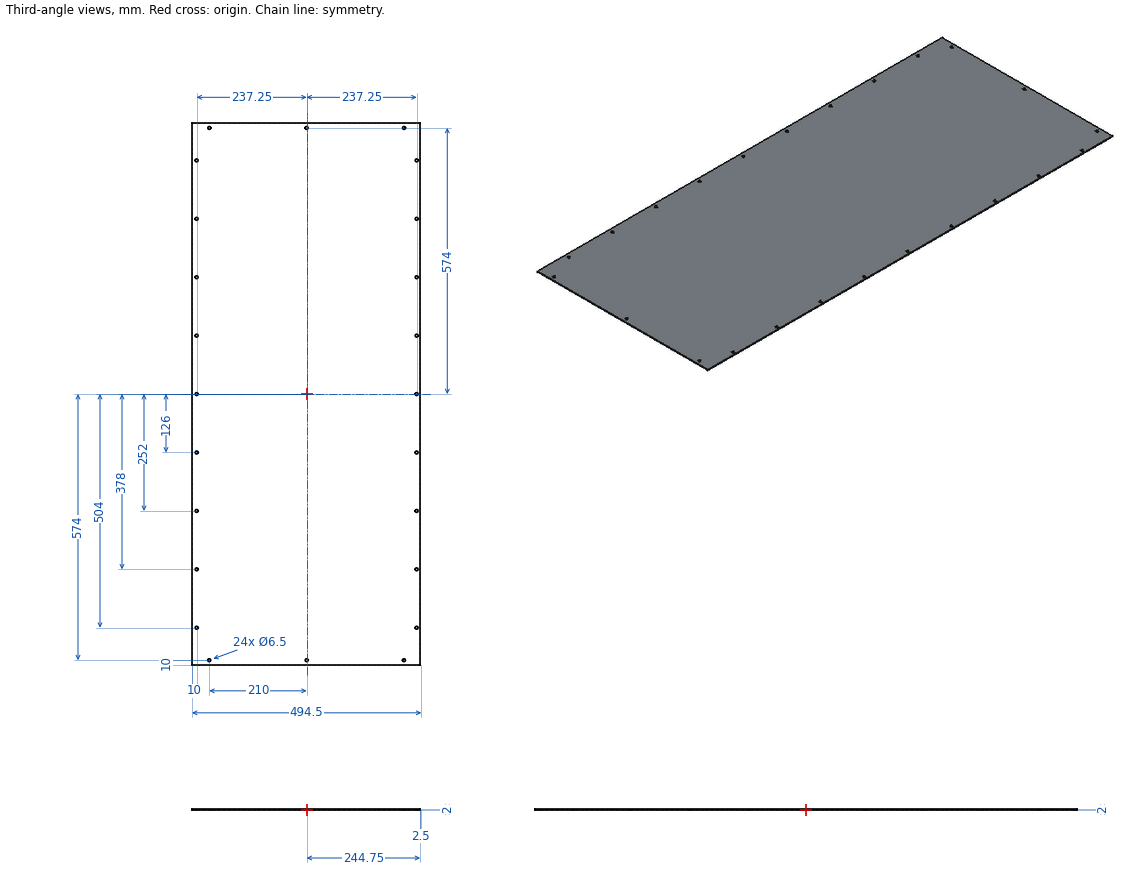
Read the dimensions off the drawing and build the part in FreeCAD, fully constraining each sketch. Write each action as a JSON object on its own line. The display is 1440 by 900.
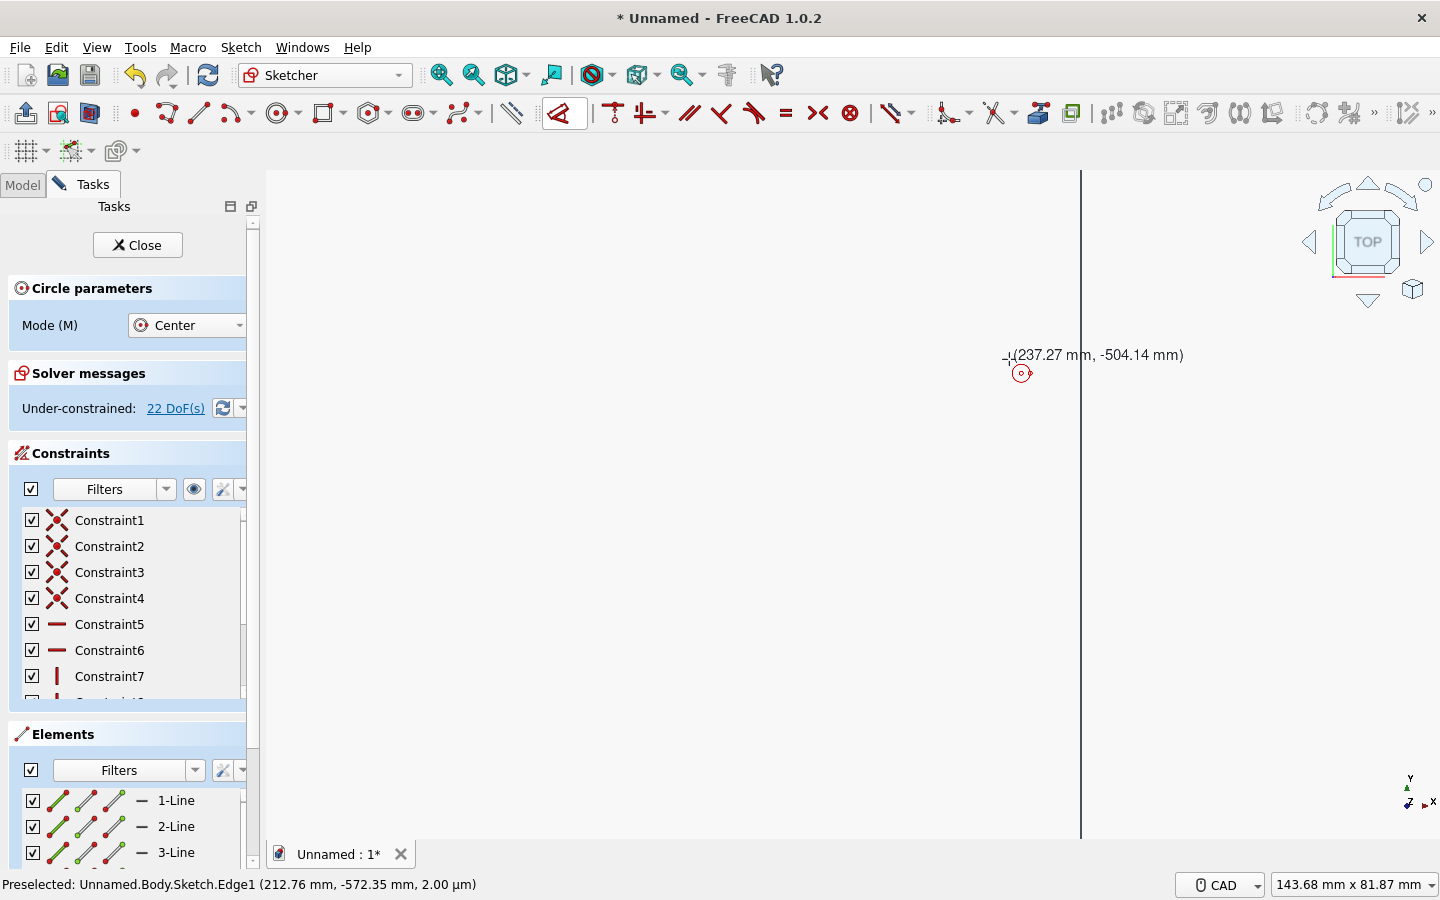
{"action": "scroll", "coordinate": [874, 728], "scroll_direction": "down", "scroll_amount": 15}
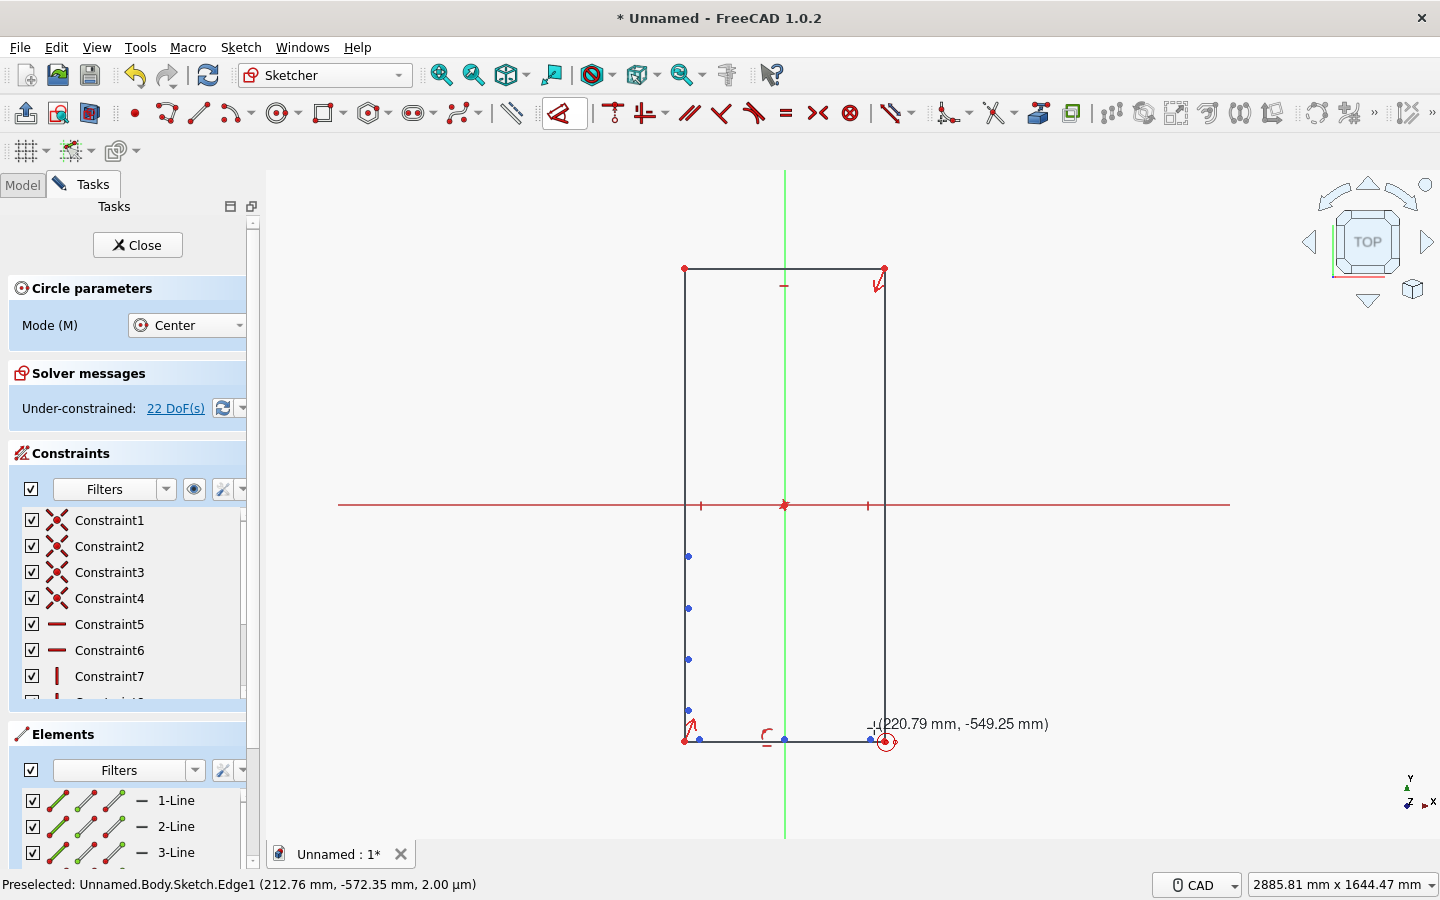
{"action": "scroll", "coordinate": [881, 710], "scroll_direction": "up", "scroll_amount": 7}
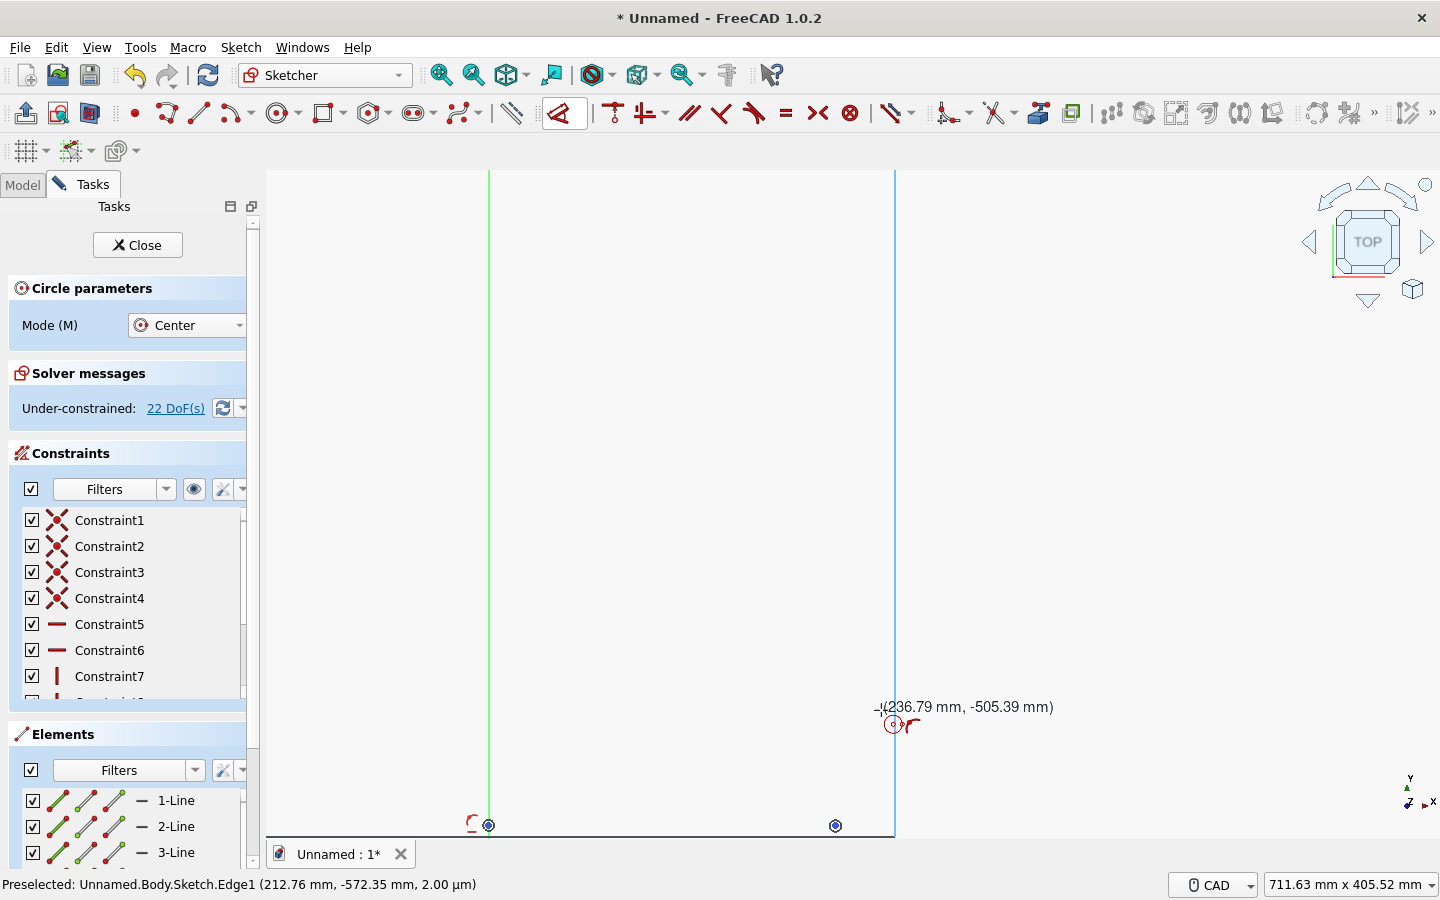
{"action": "left_click", "coordinate": [880, 709]}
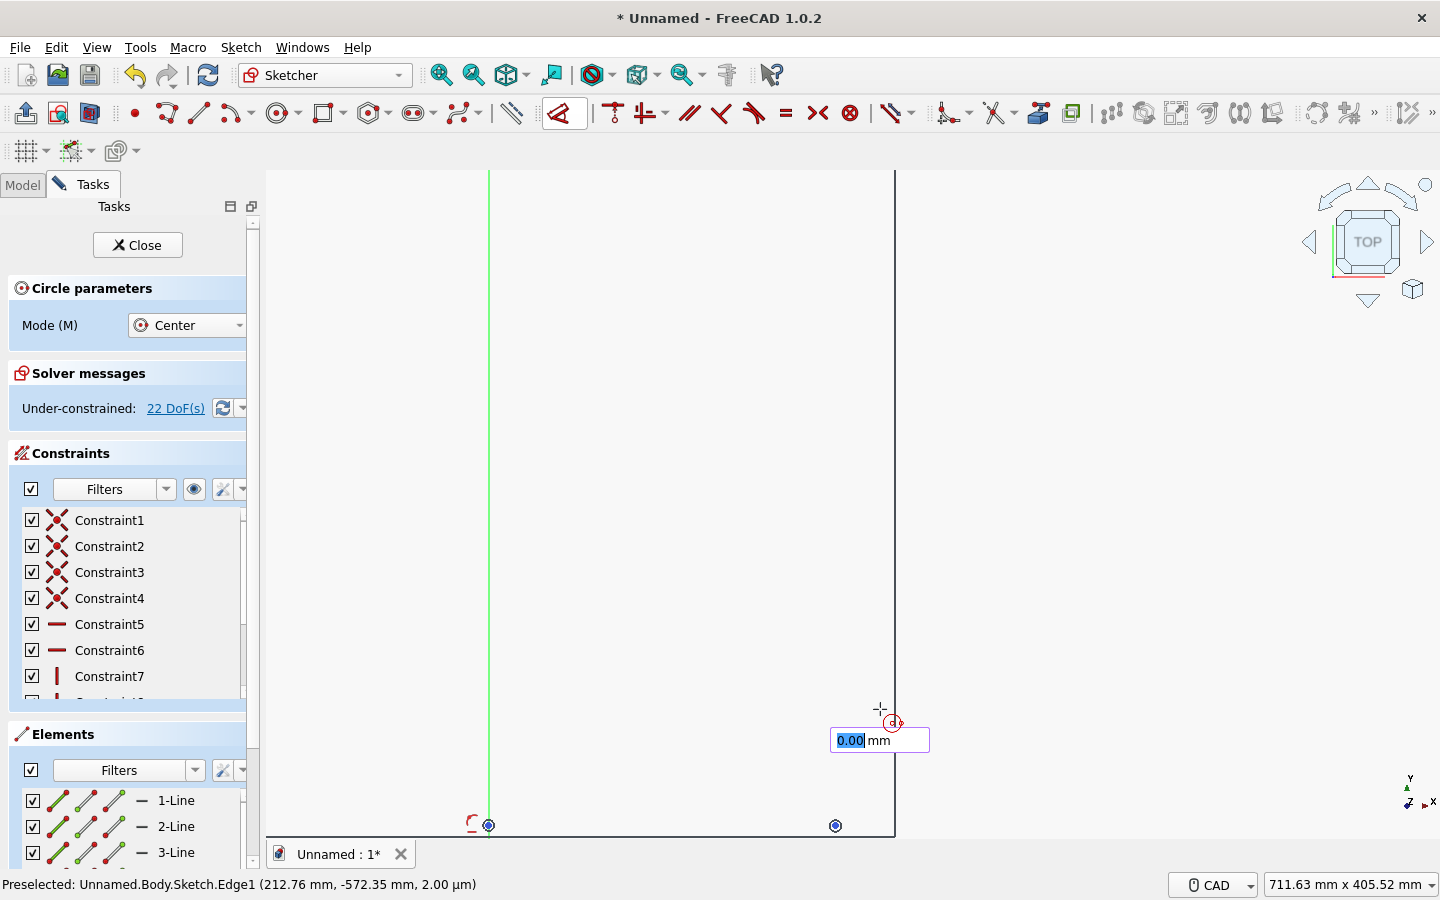
{"action": "scroll", "coordinate": [876, 705], "scroll_direction": "up", "scroll_amount": 6}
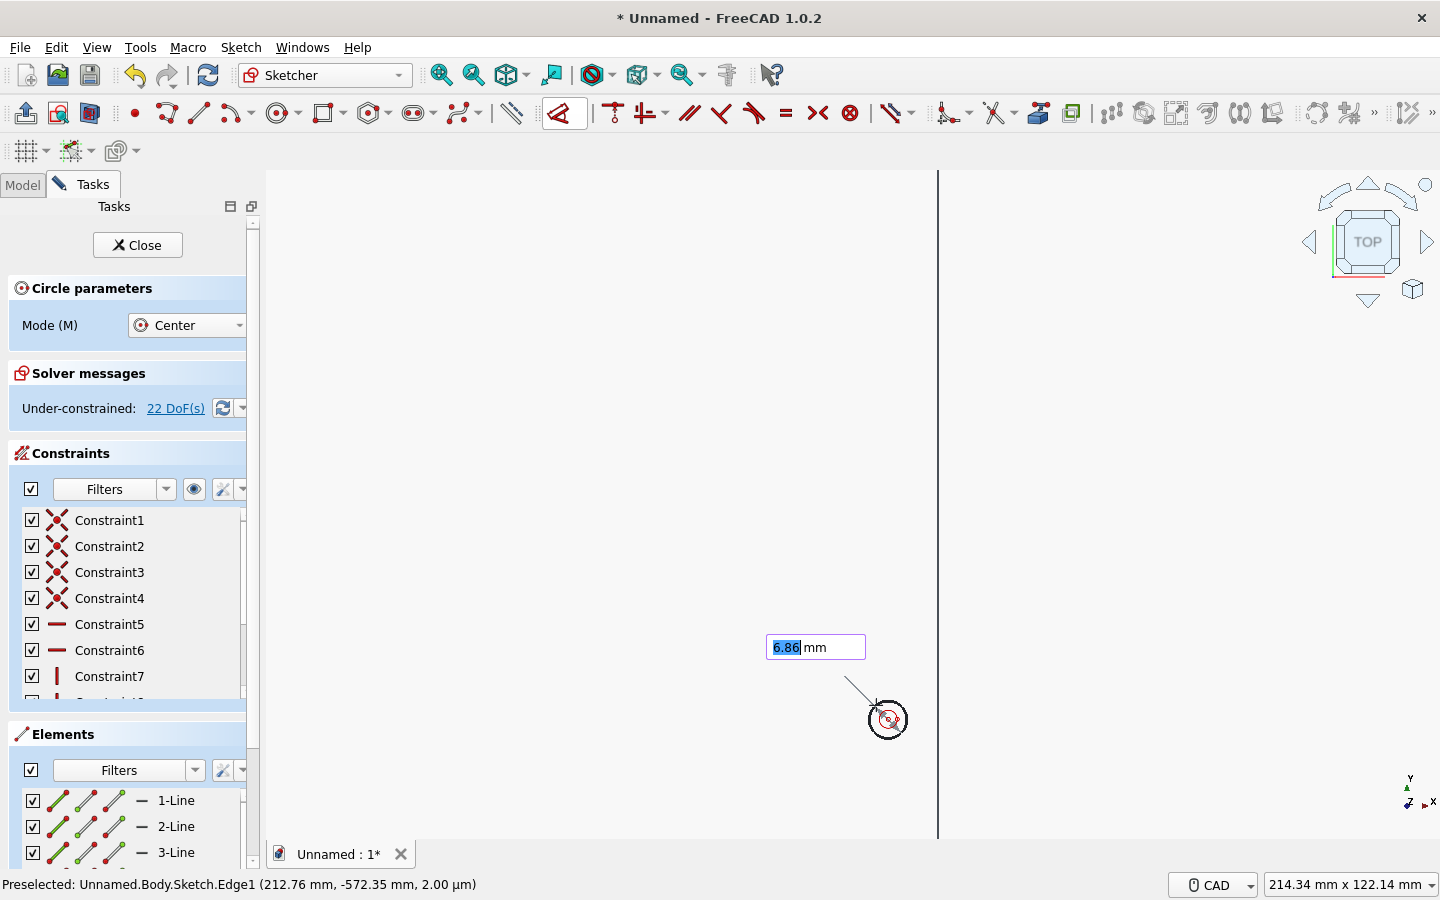
{"action": "left_click", "coordinate": [876, 705]}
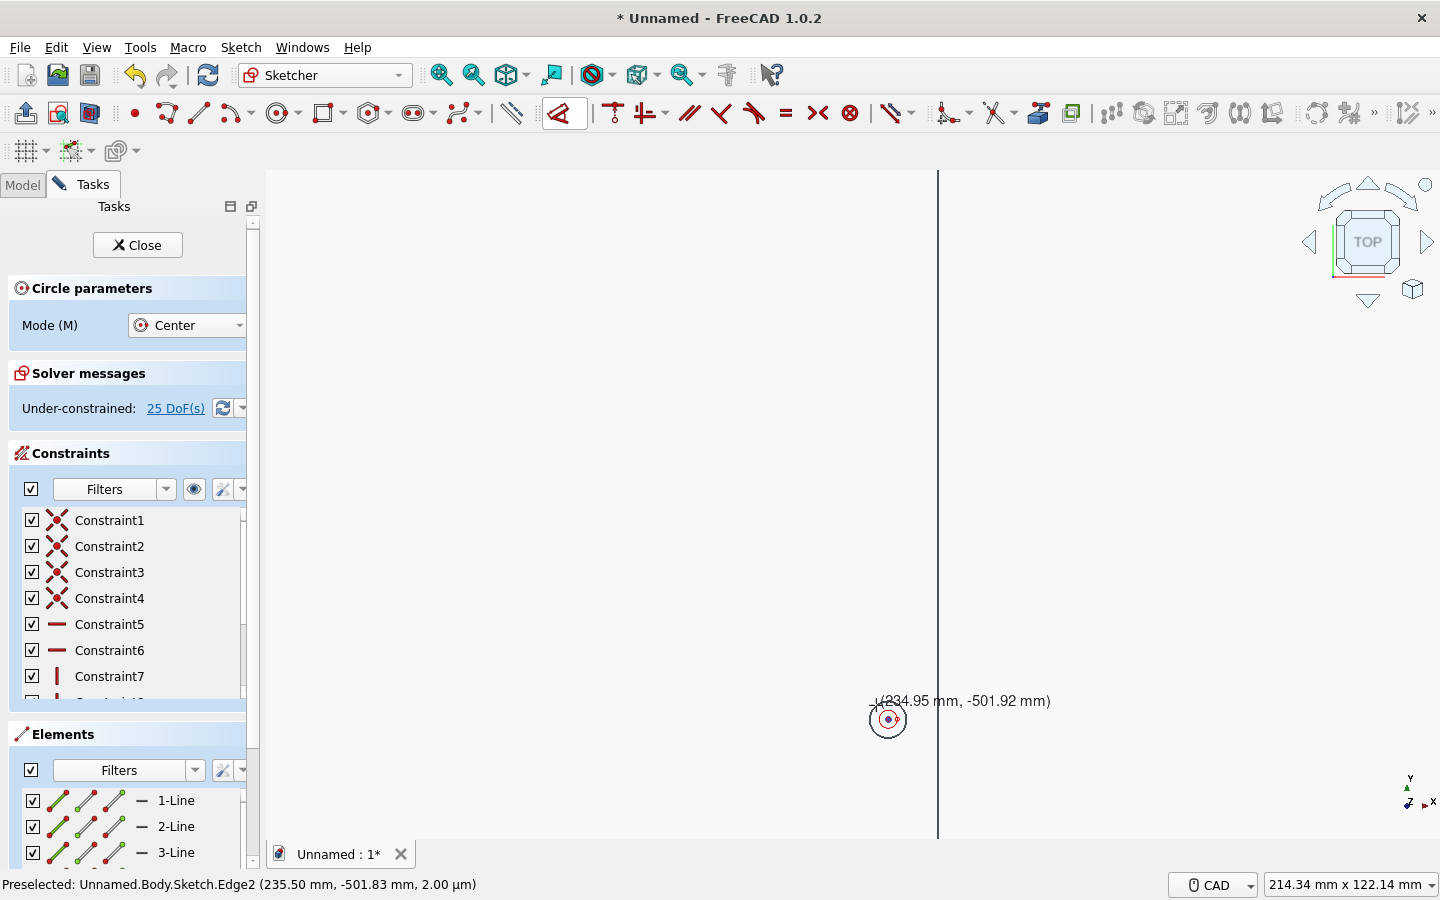
{"action": "scroll", "coordinate": [880, 709], "scroll_direction": "down", "scroll_amount": 13}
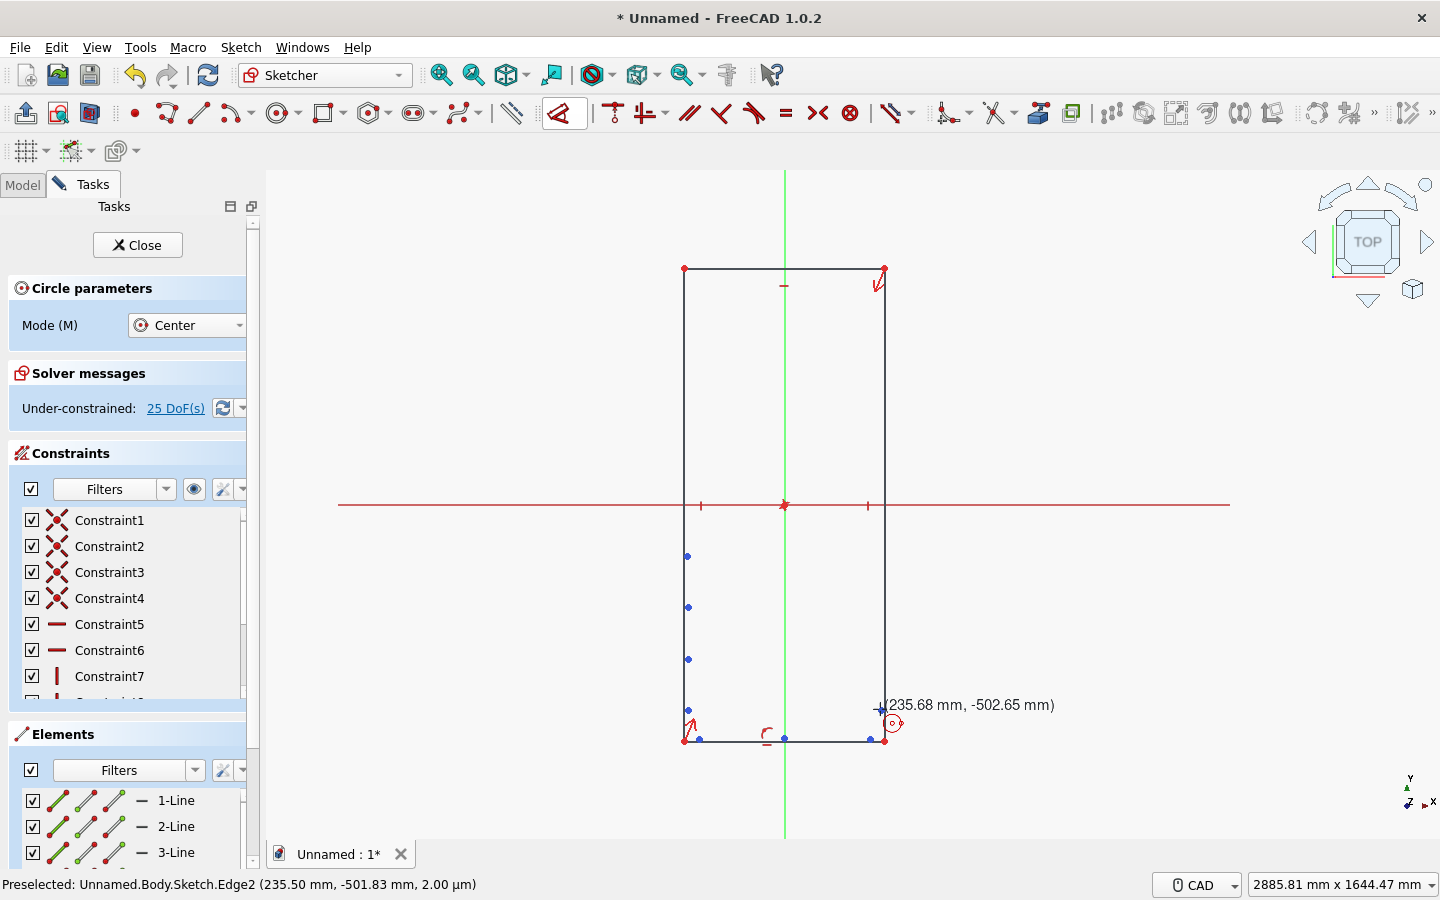
{"action": "scroll", "coordinate": [881, 659], "scroll_direction": "up", "scroll_amount": 15}